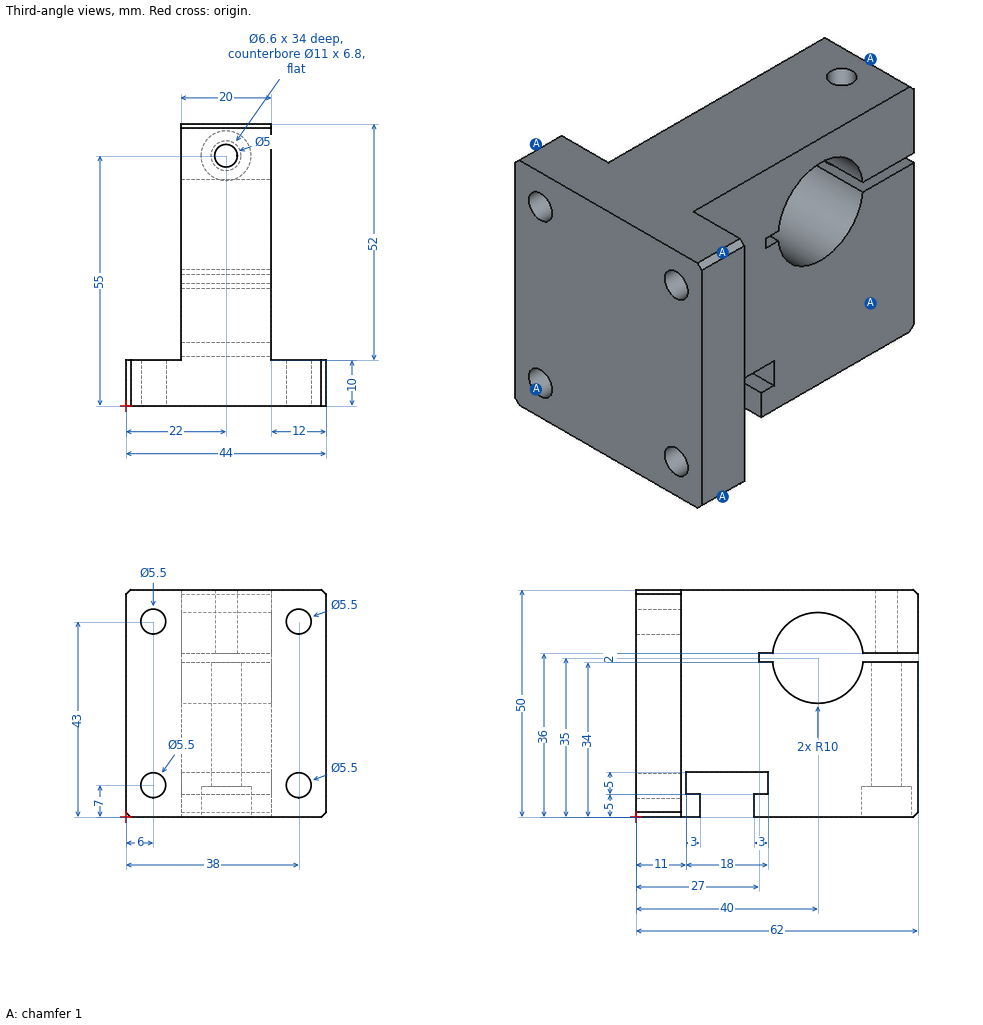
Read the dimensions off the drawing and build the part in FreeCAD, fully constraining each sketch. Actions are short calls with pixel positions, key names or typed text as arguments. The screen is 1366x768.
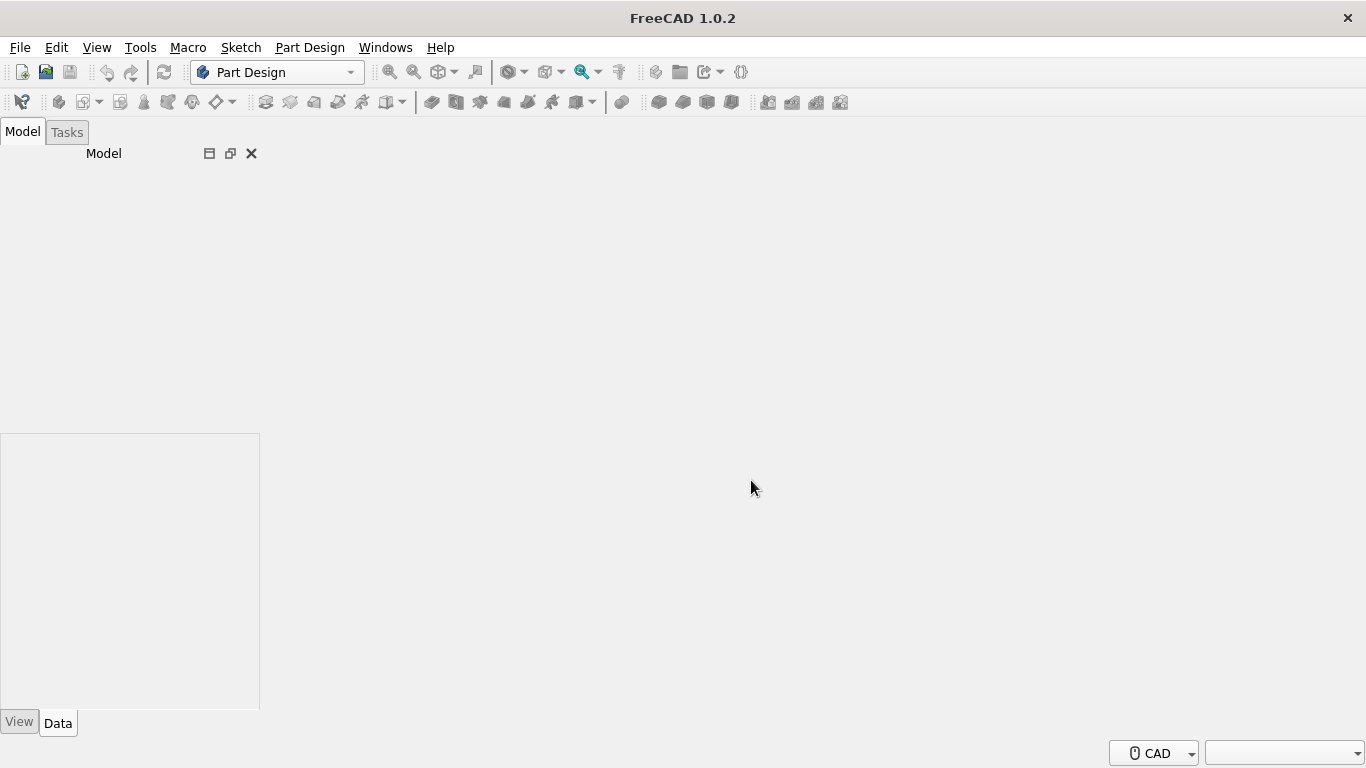
click(22, 72)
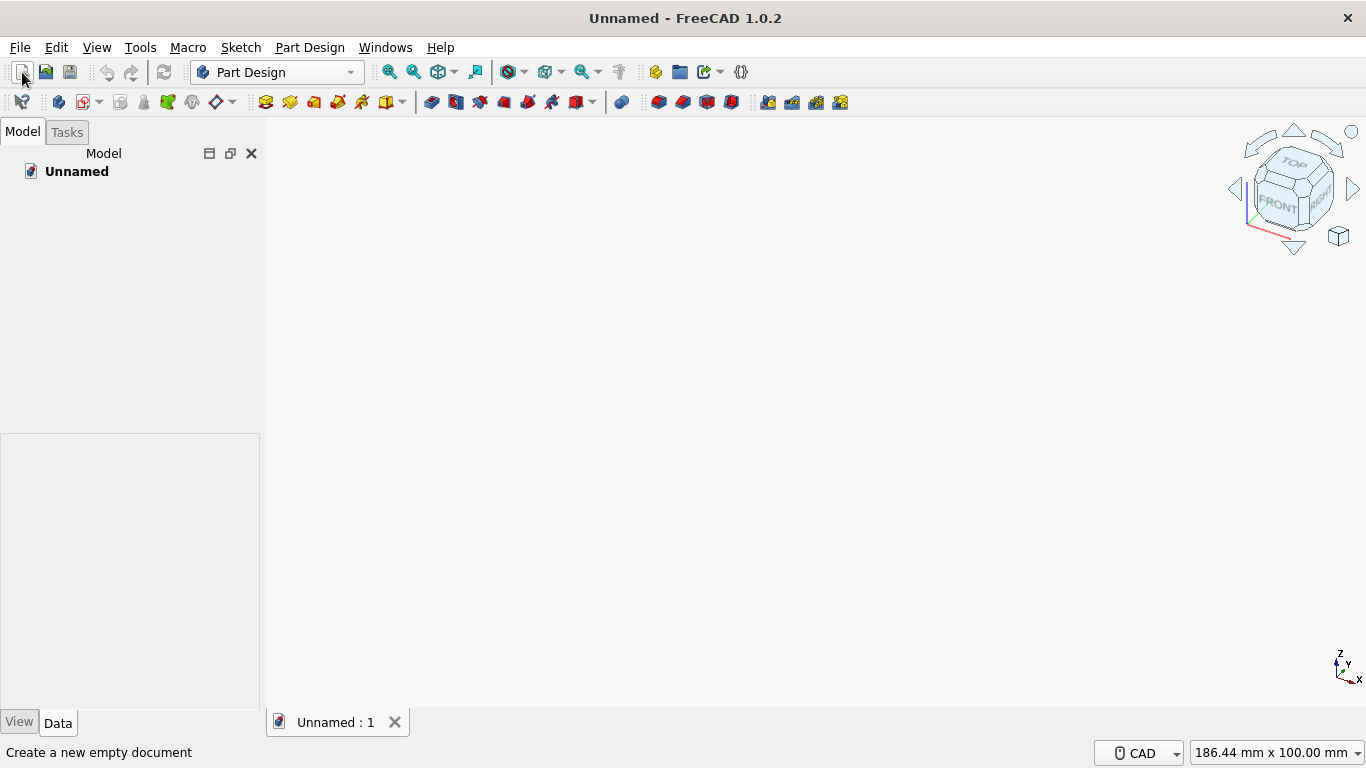
click(84, 102)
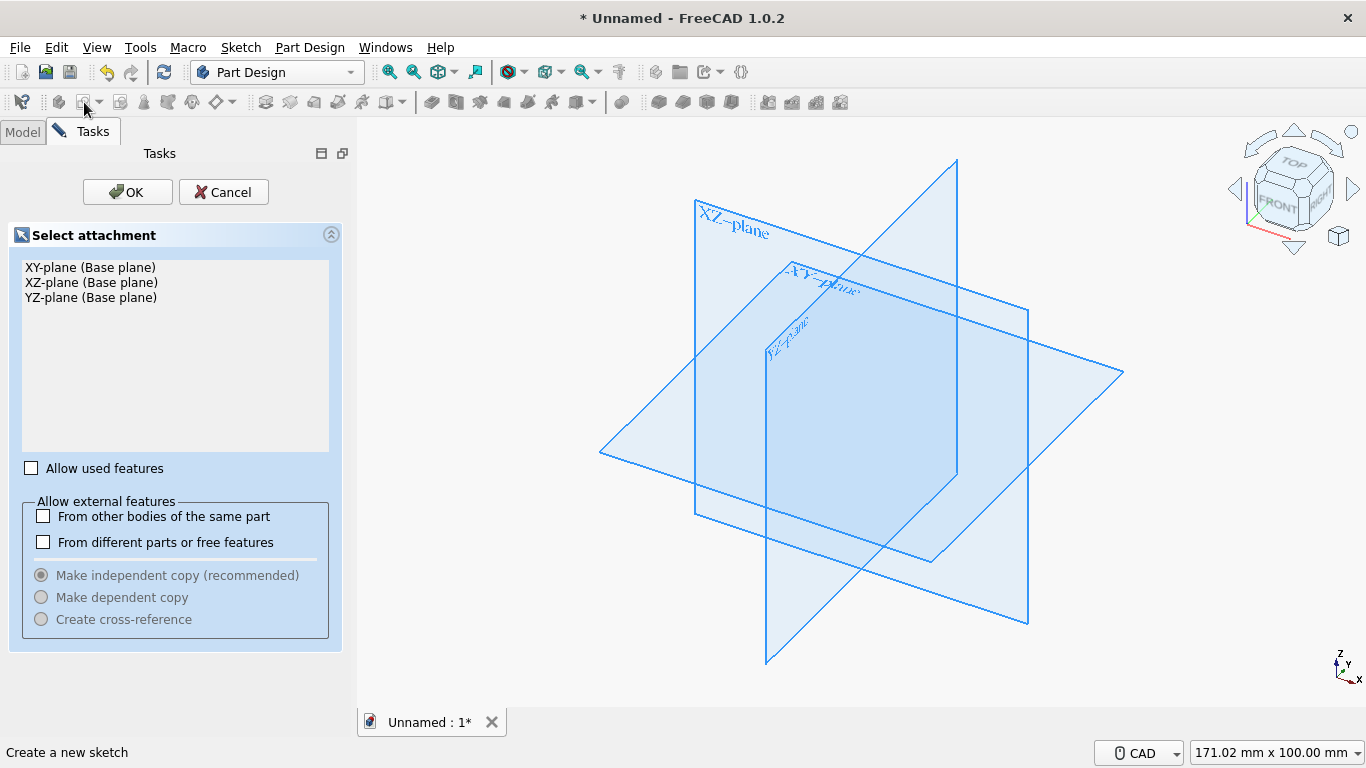
click(82, 268)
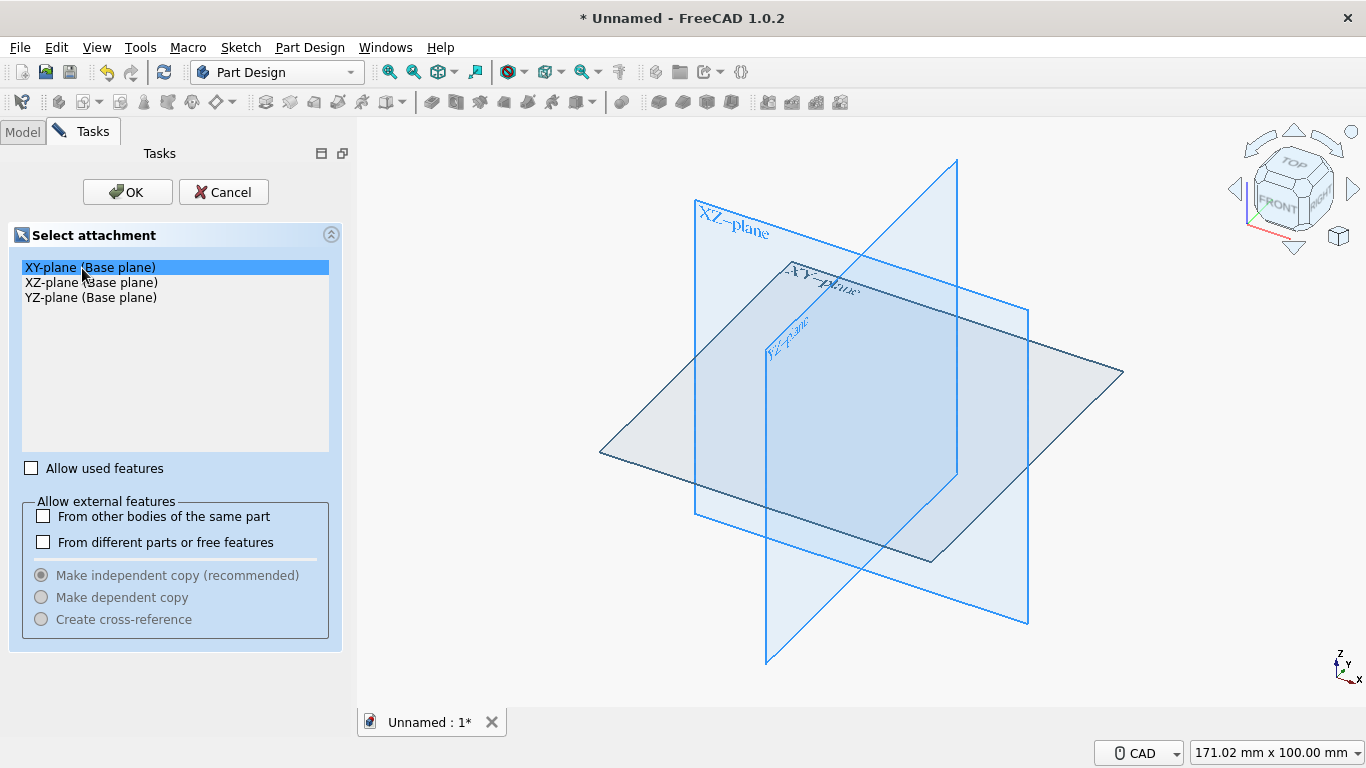
click(128, 192)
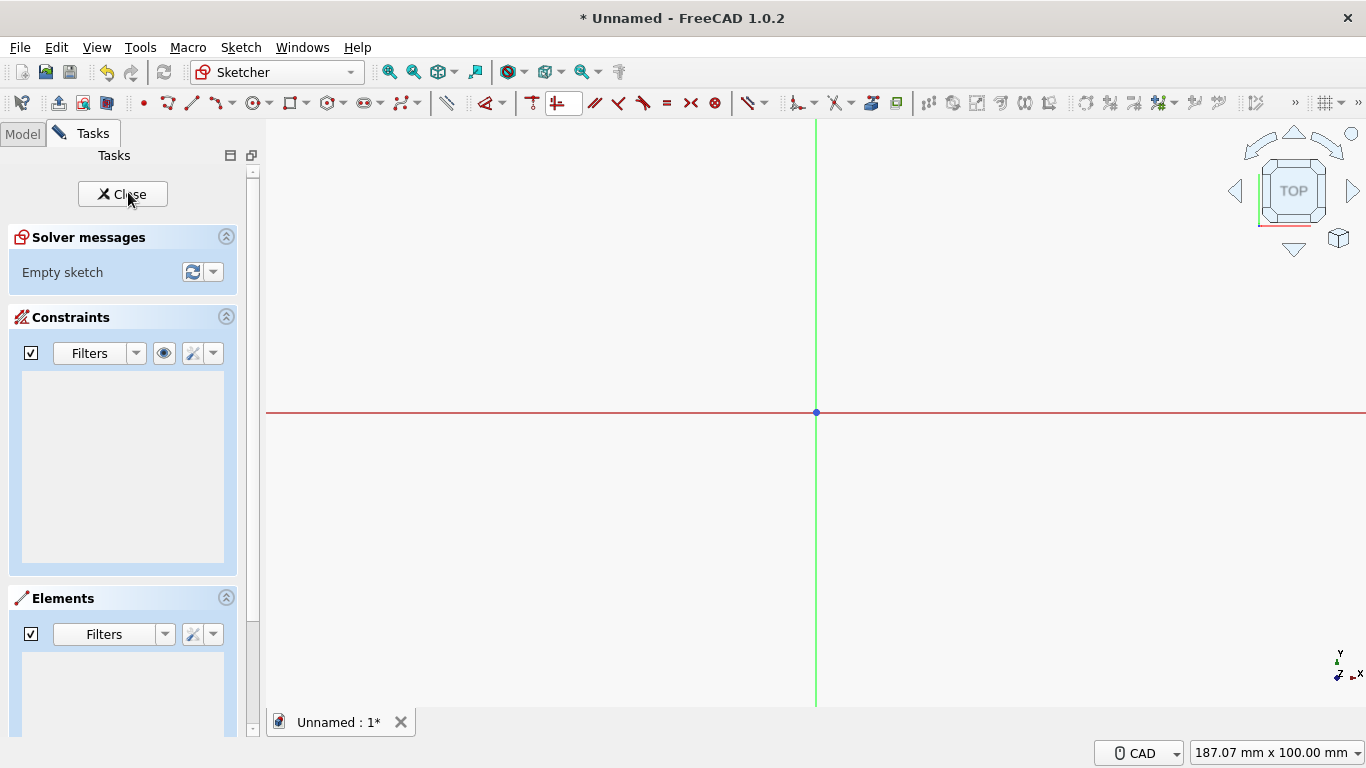
scroll(345, 679, down, 2)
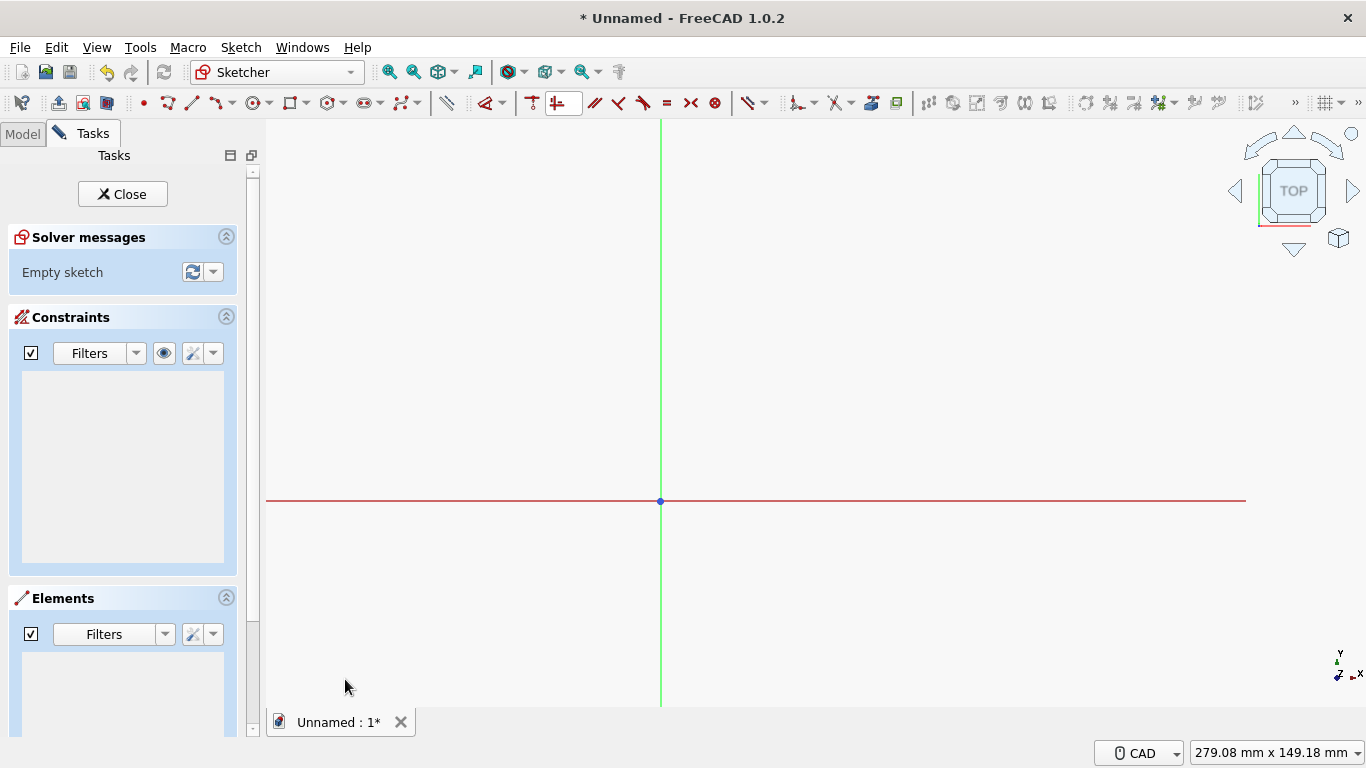
scroll(747, 309, up, 2)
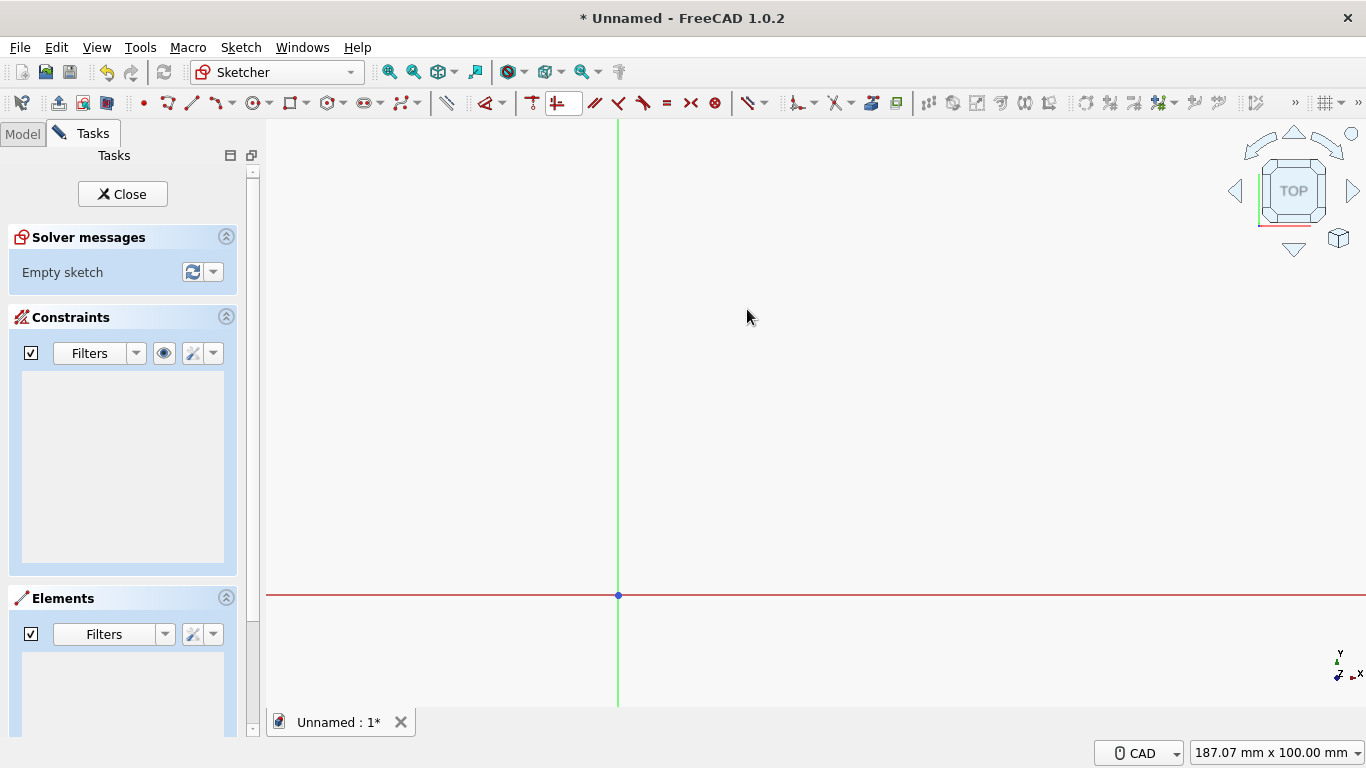
click(168, 104)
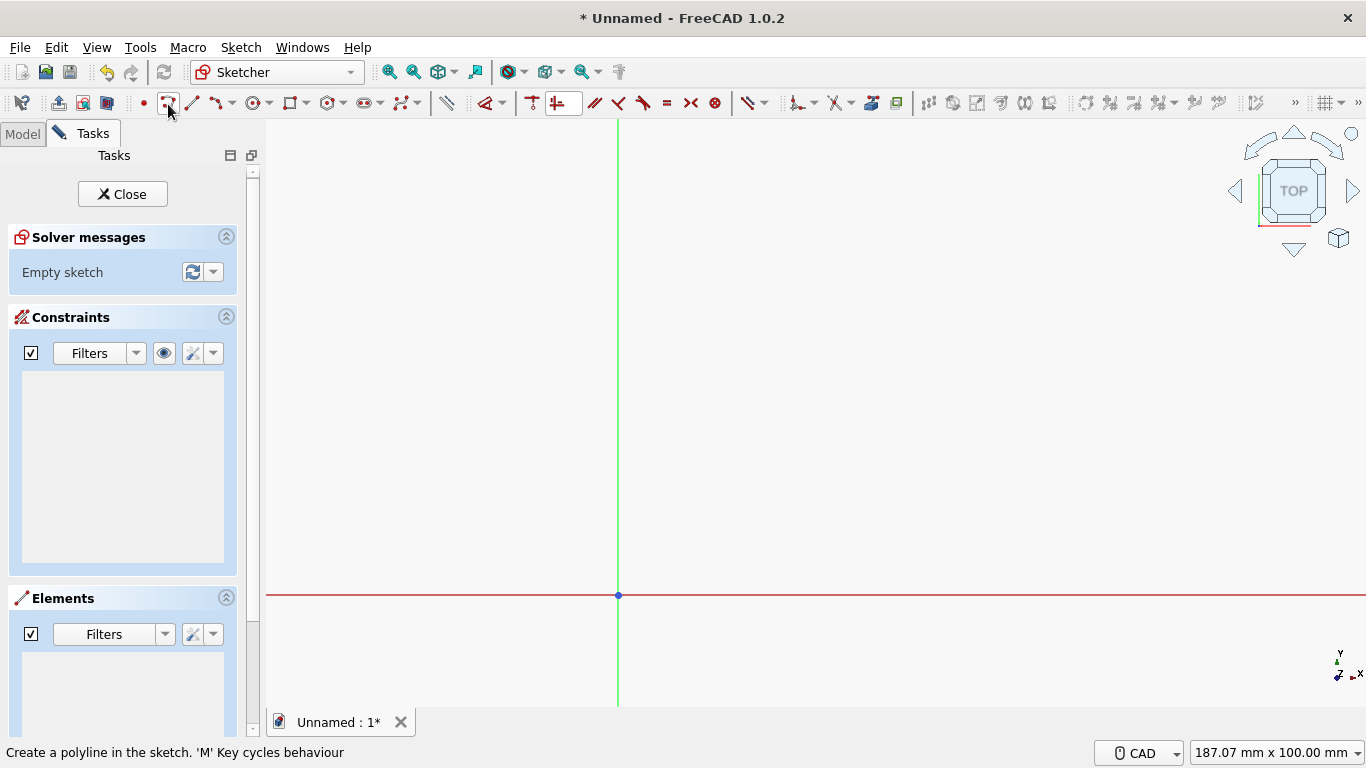
click(618, 595)
click(877, 586)
click(877, 536)
click(806, 536)
click(806, 231)
click(689, 231)
click(689, 536)
click(627, 536)
click(618, 595)
key(Escape)
key(Escape)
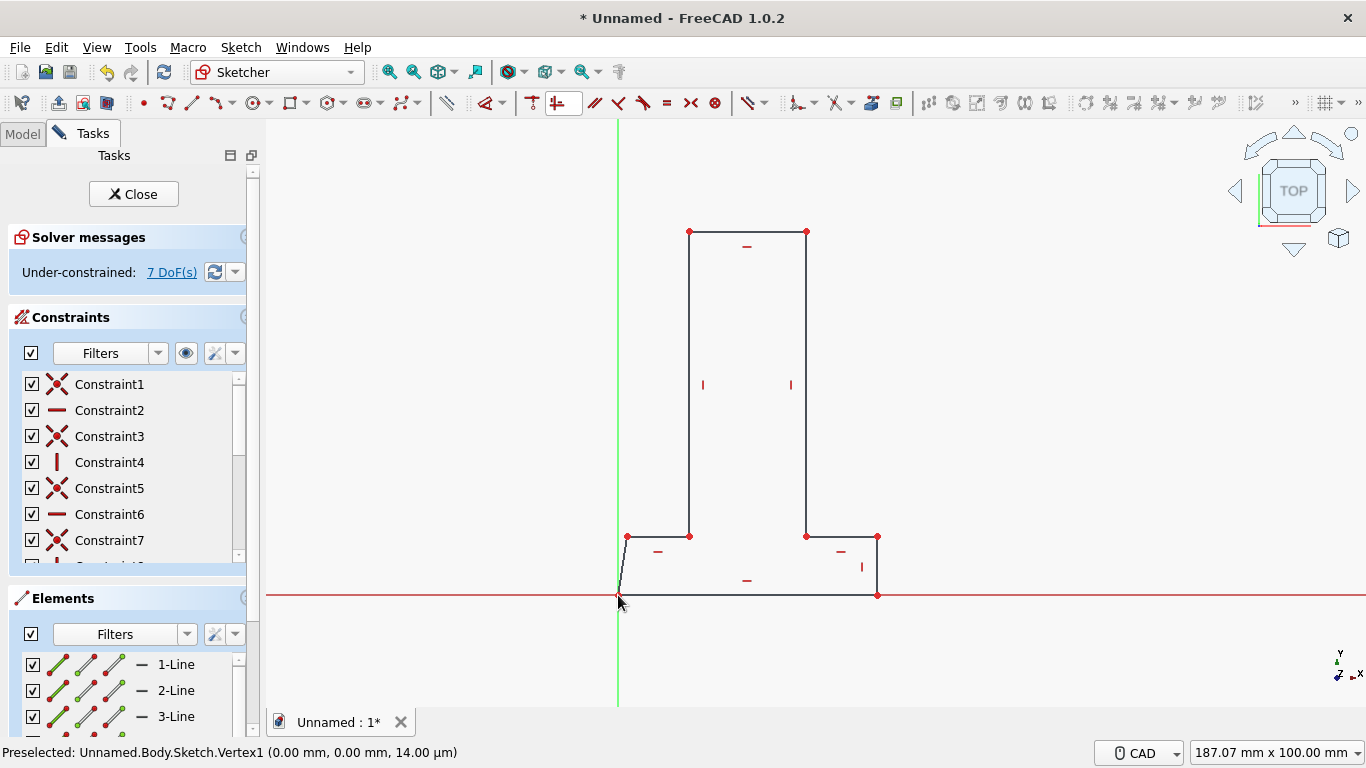
click(621, 578)